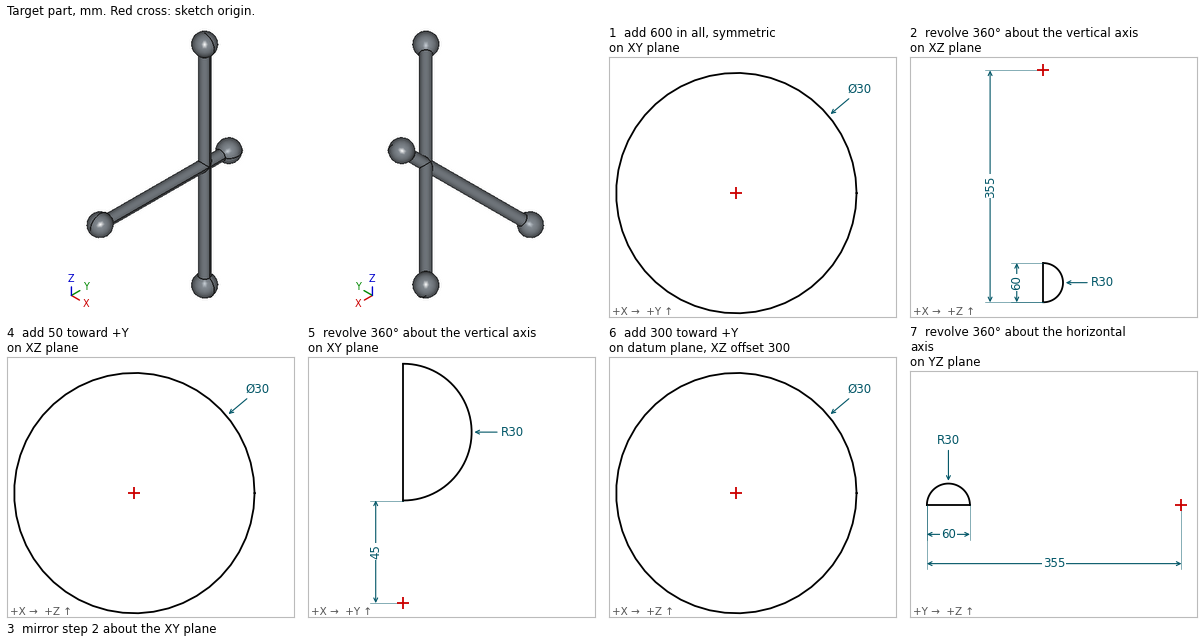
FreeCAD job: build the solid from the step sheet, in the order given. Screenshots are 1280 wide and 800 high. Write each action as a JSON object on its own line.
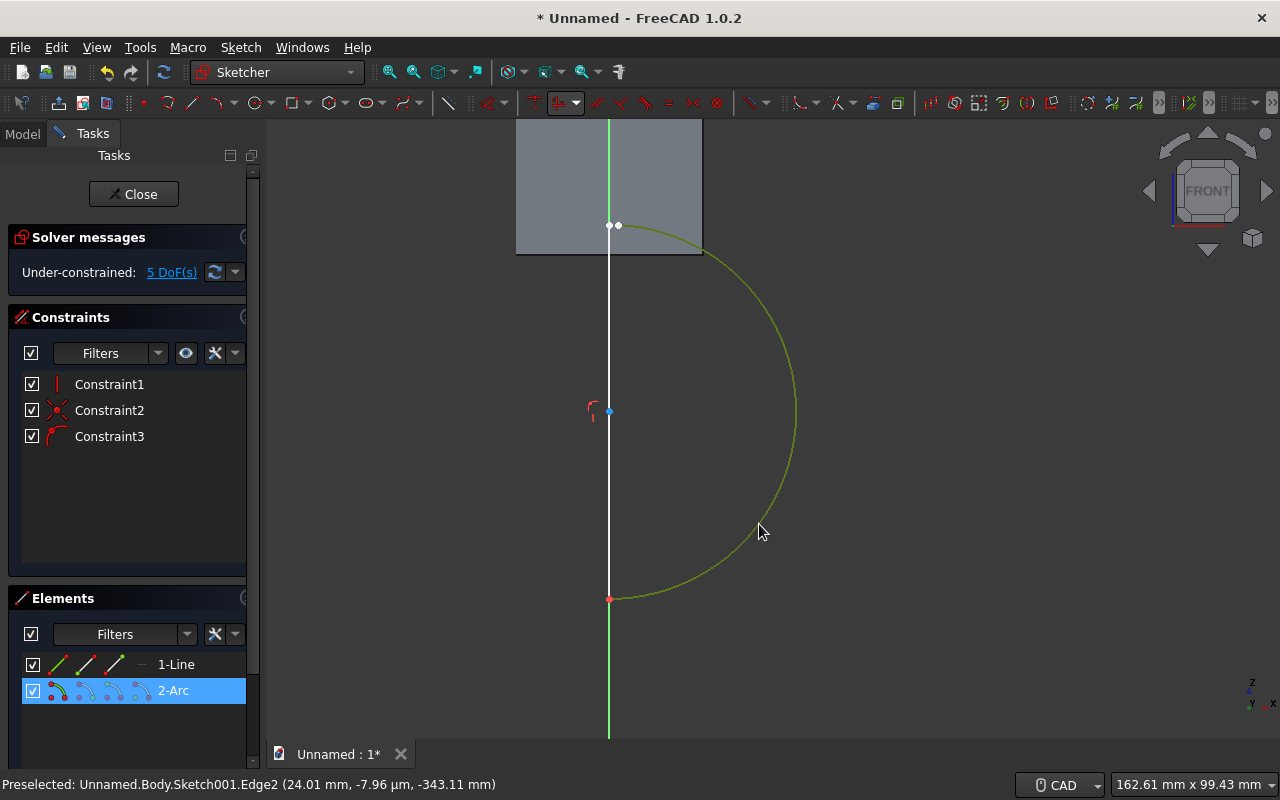
{"action": "left_click", "coordinate": [506, 104]}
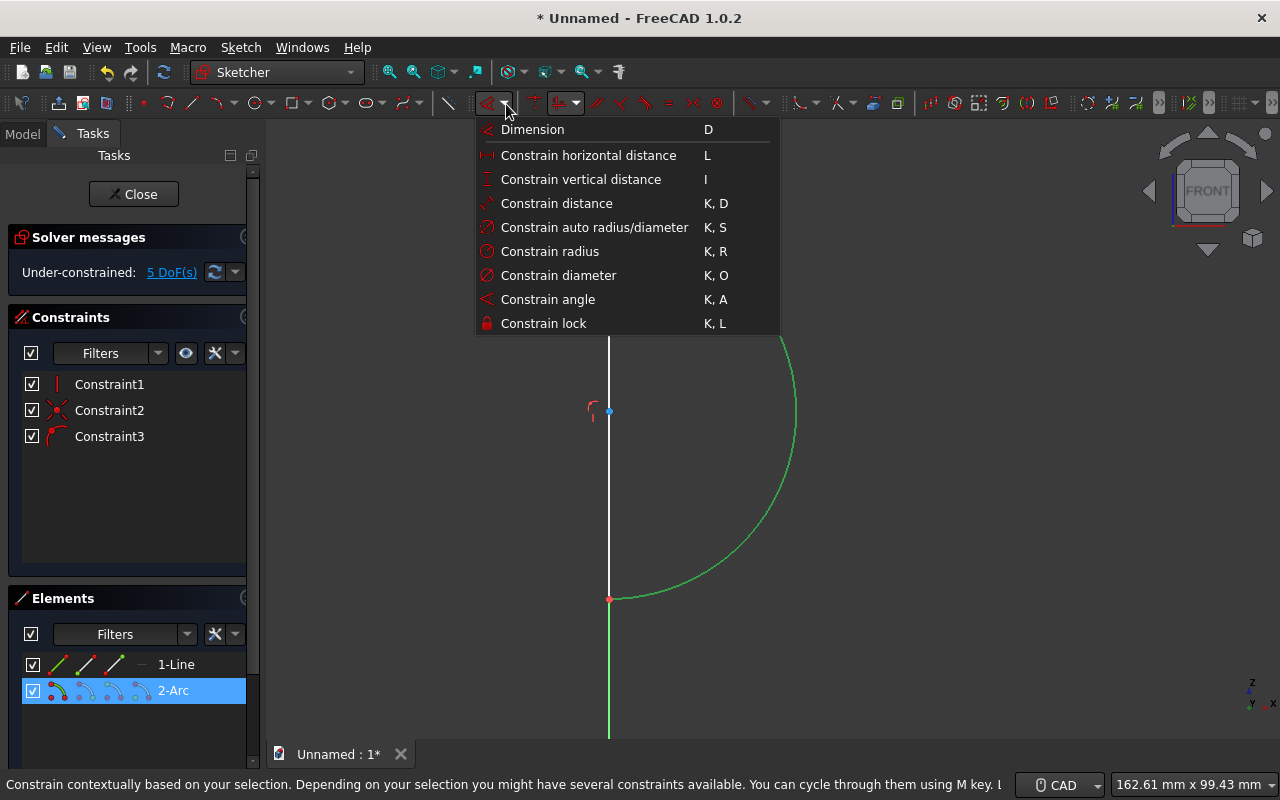
{"action": "left_click", "coordinate": [628, 251]}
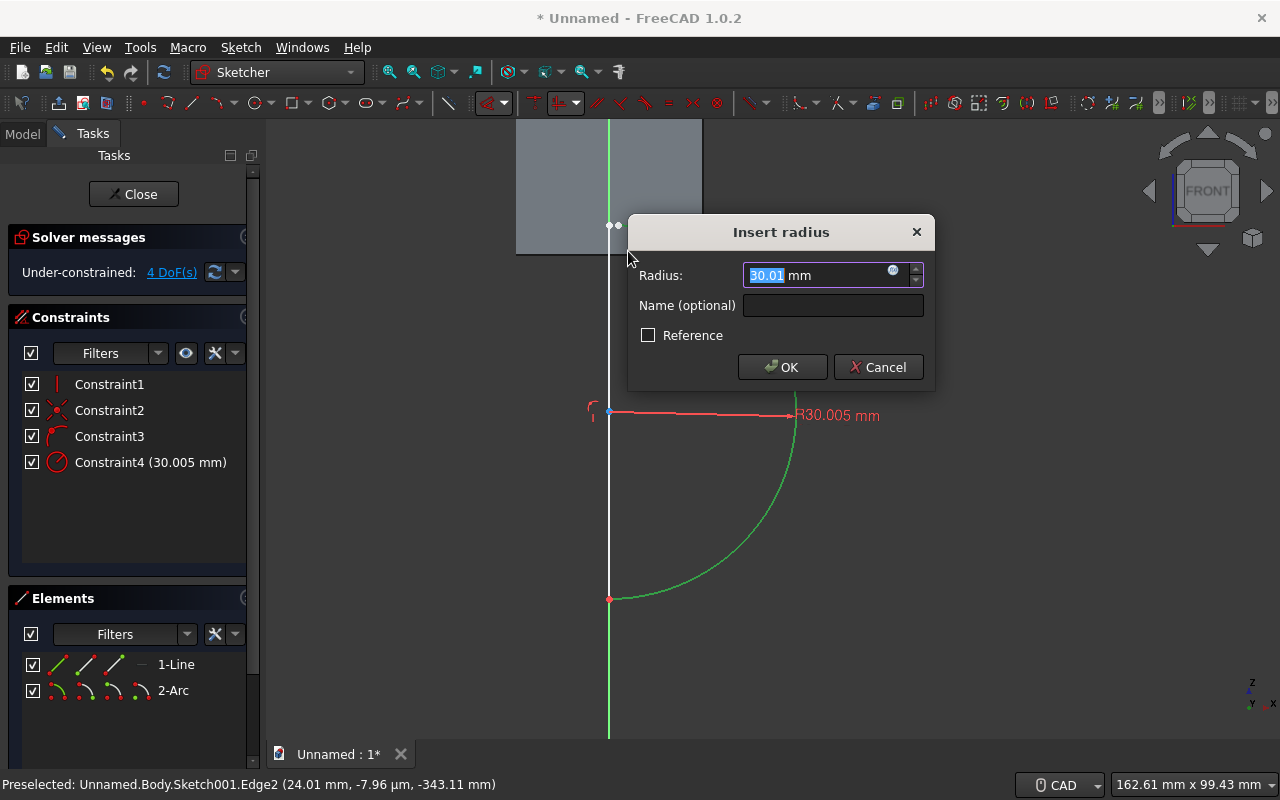
{"action": "type", "text": "30"}
{"action": "key", "text": "Return"}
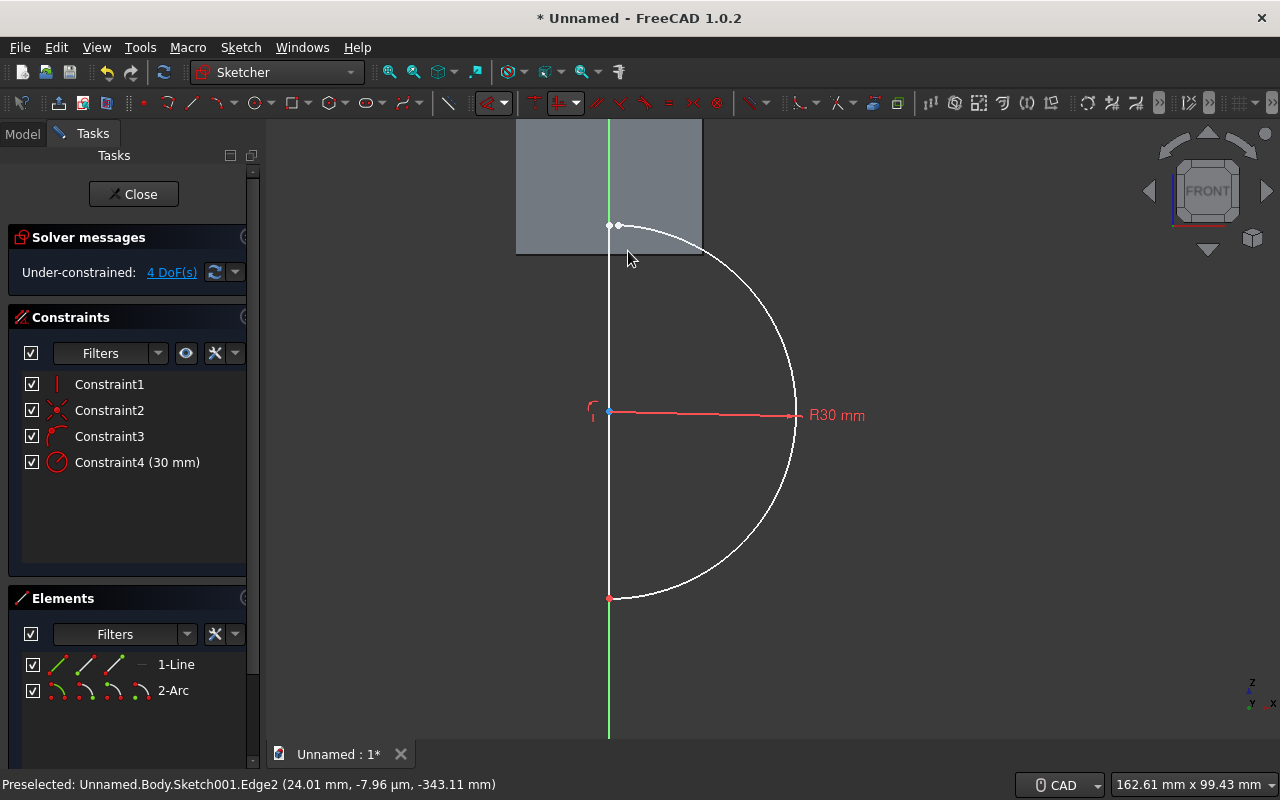
{"action": "left_click", "coordinate": [609, 599]}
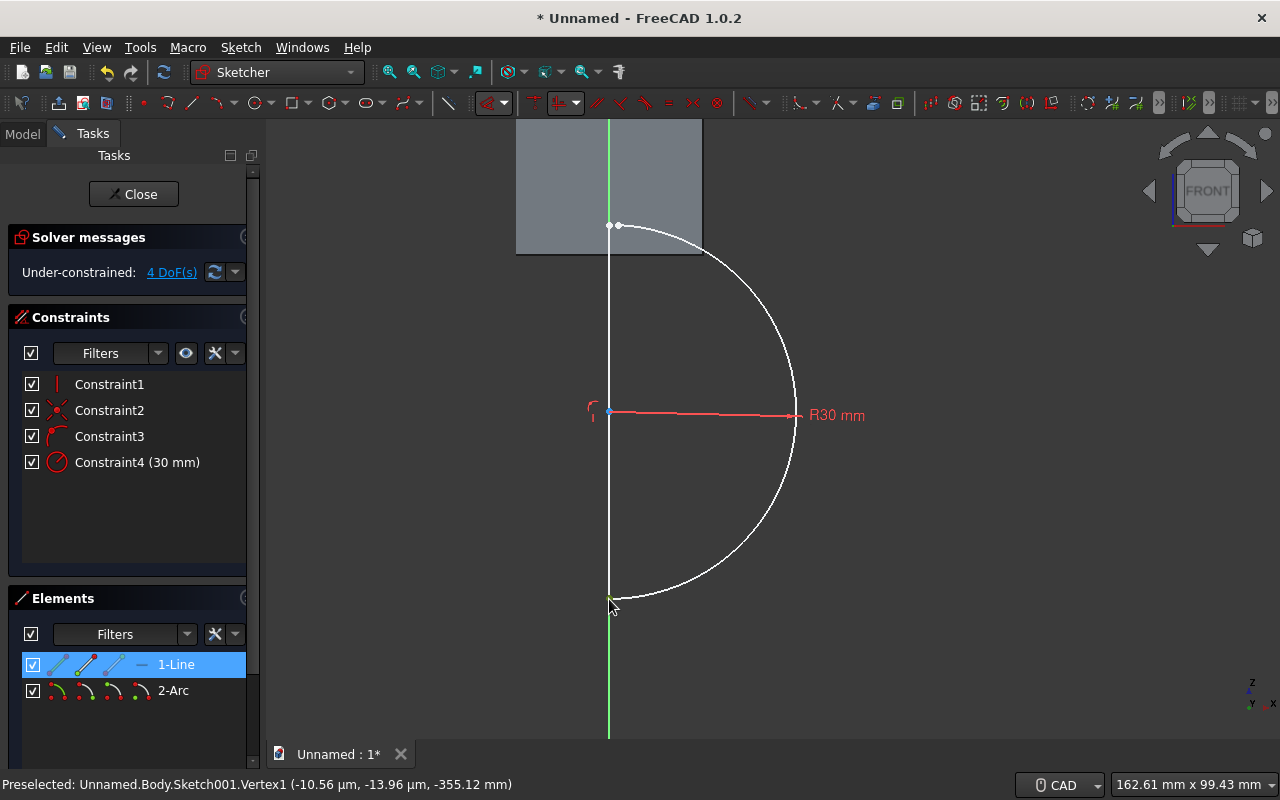
{"action": "left_click", "coordinate": [609, 671]}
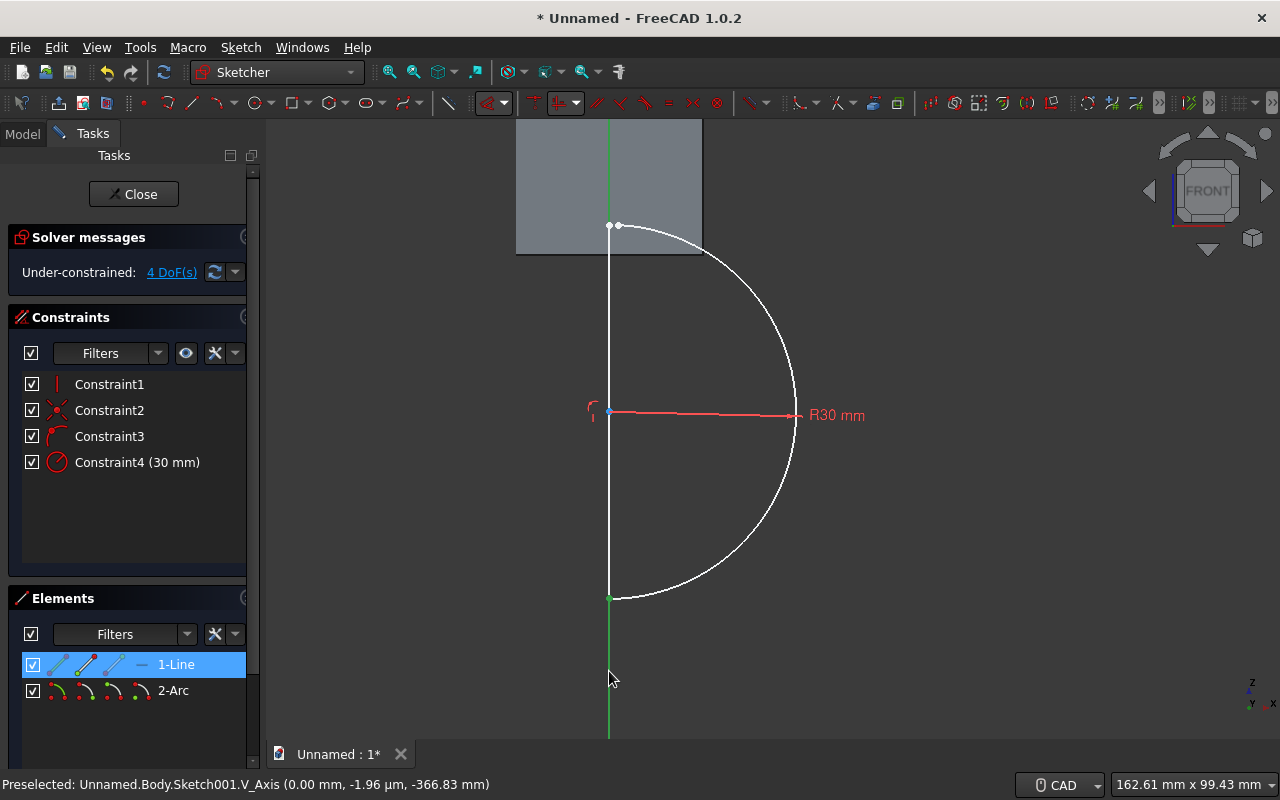
{"action": "left_click", "coordinate": [534, 104]}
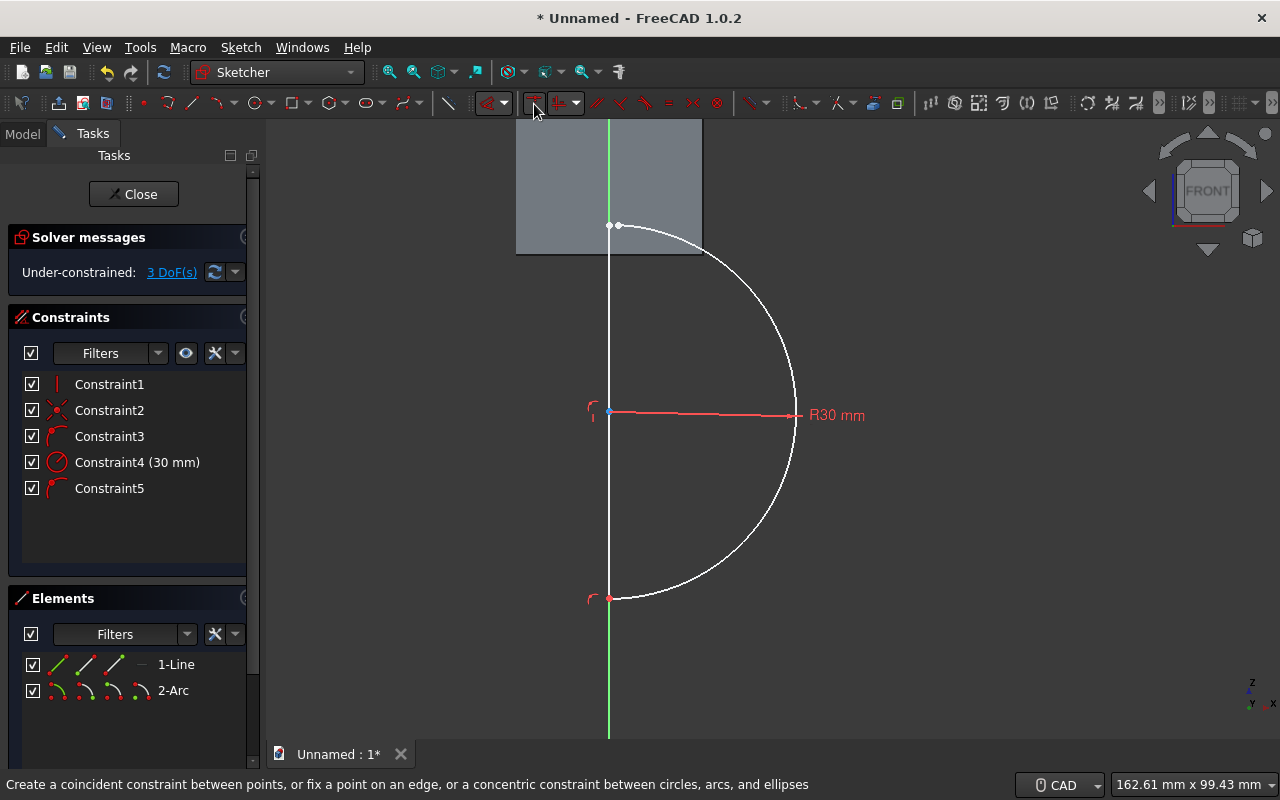
{"action": "left_click", "coordinate": [618, 225]}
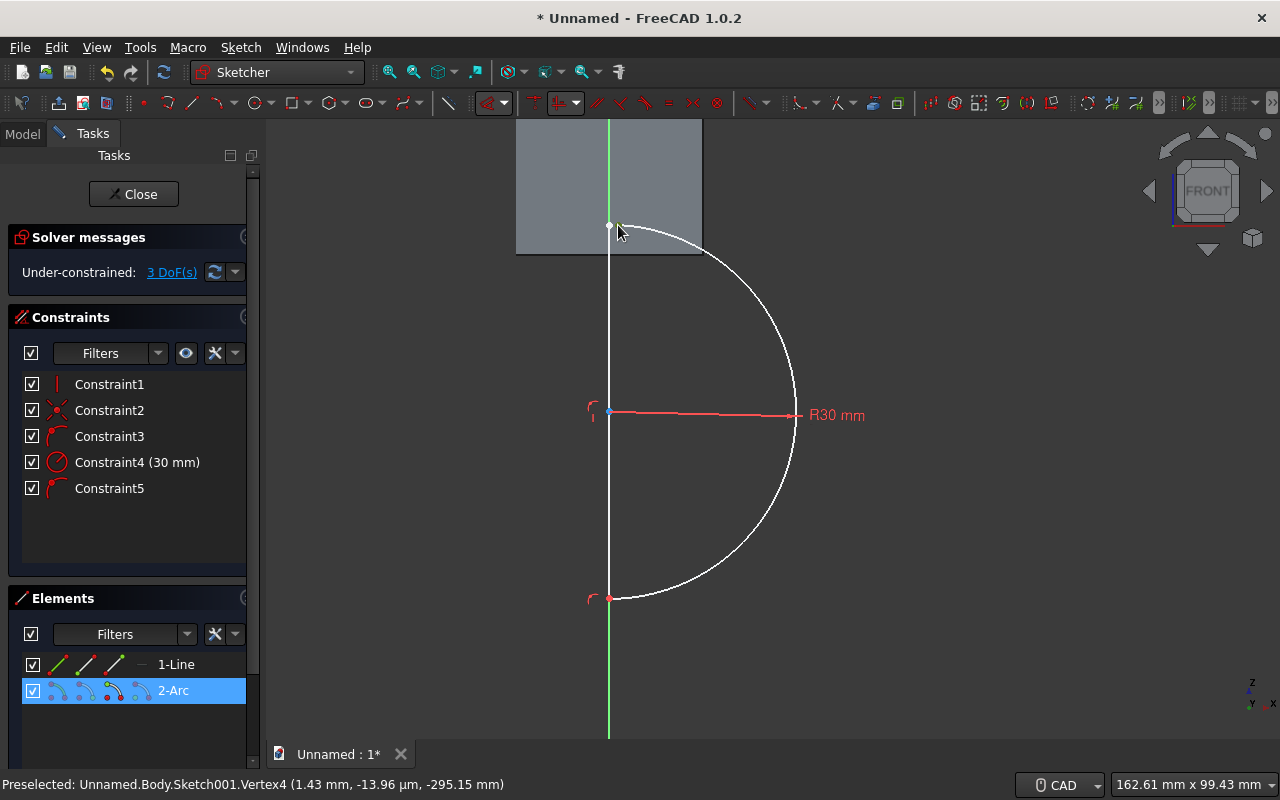
{"action": "left_click", "coordinate": [609, 671]}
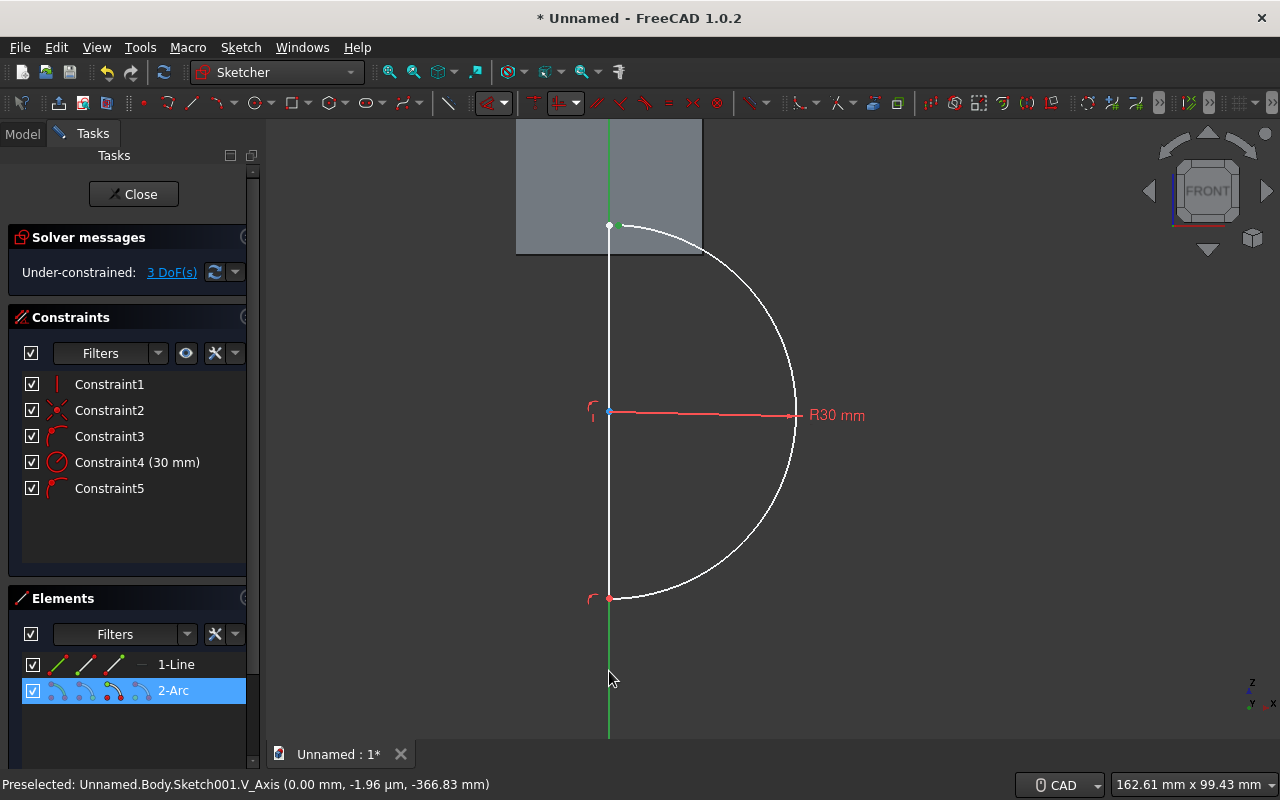
{"action": "left_click", "coordinate": [534, 104]}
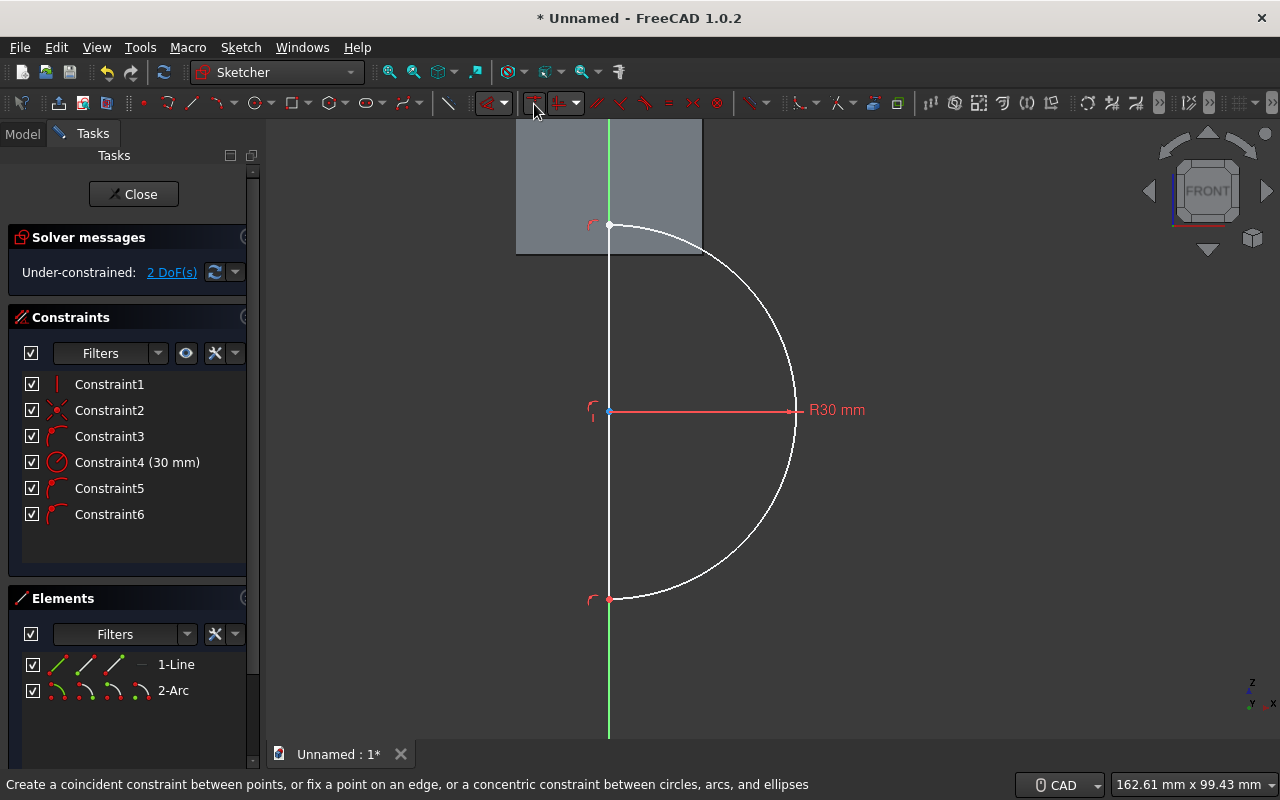
{"action": "left_click", "coordinate": [609, 487]}